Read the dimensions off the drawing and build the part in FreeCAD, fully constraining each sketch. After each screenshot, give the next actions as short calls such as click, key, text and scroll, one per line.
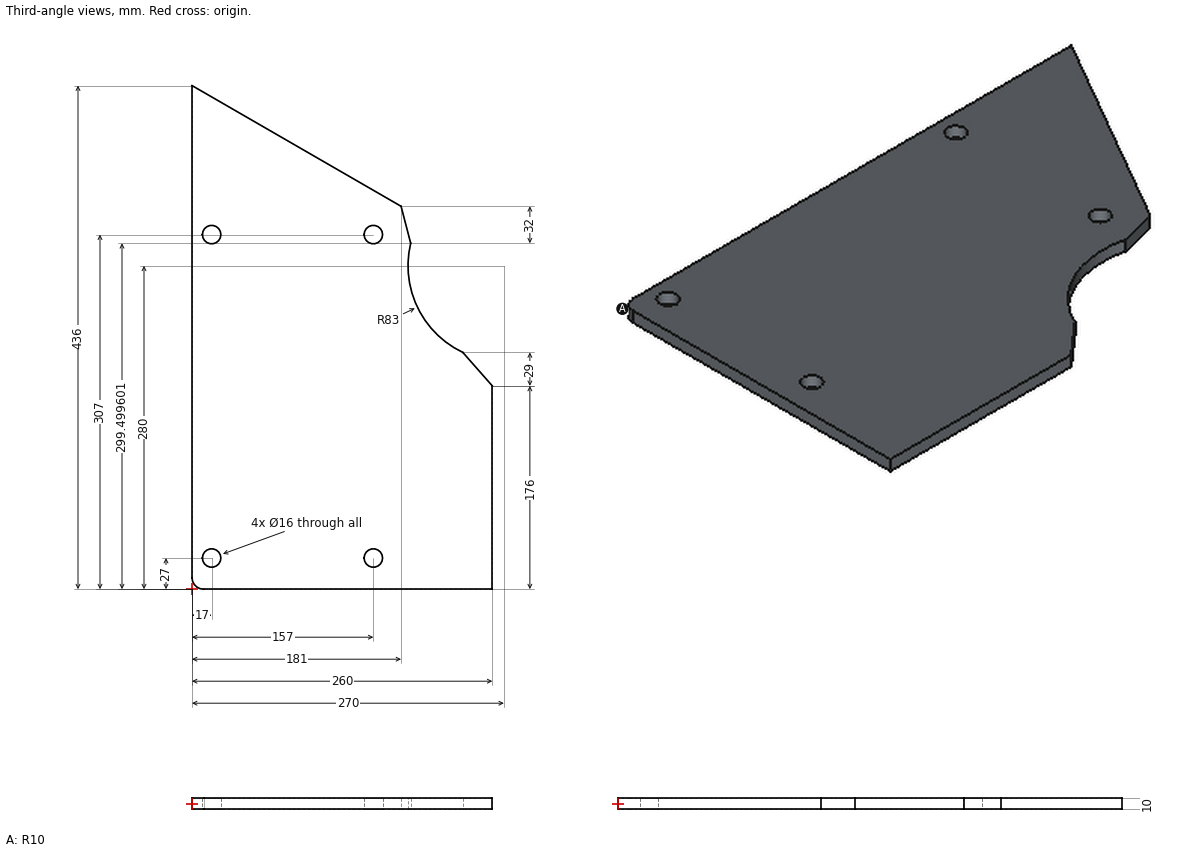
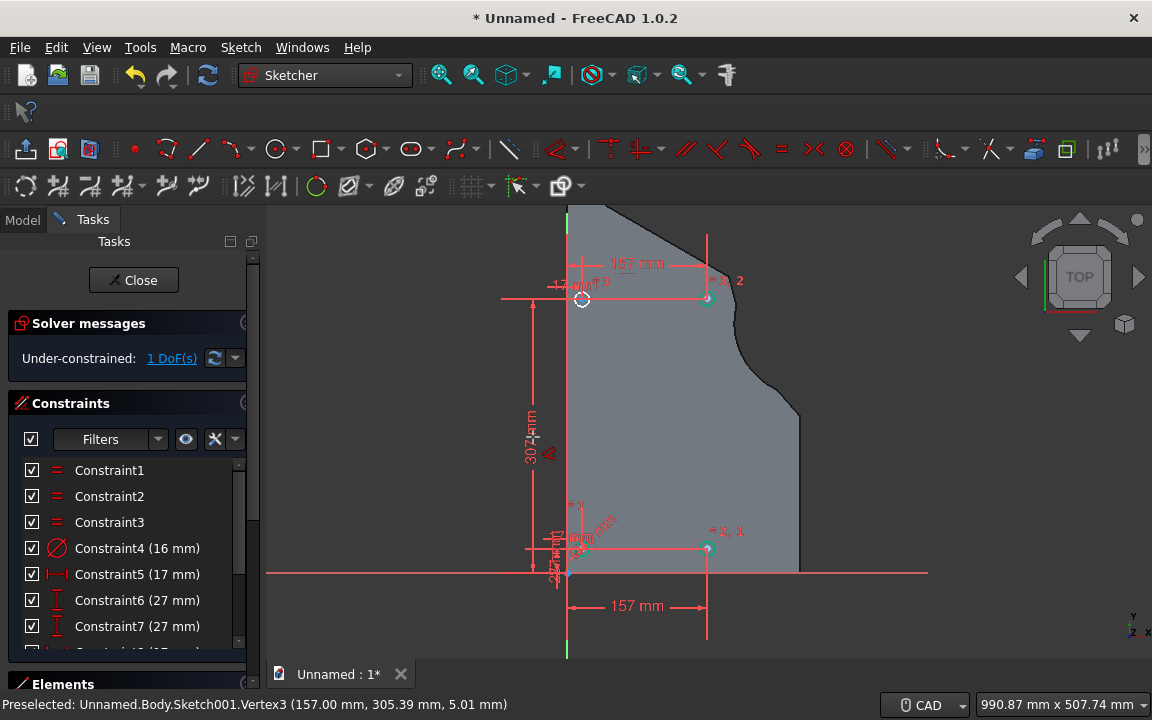
click(582, 299)
click(533, 373)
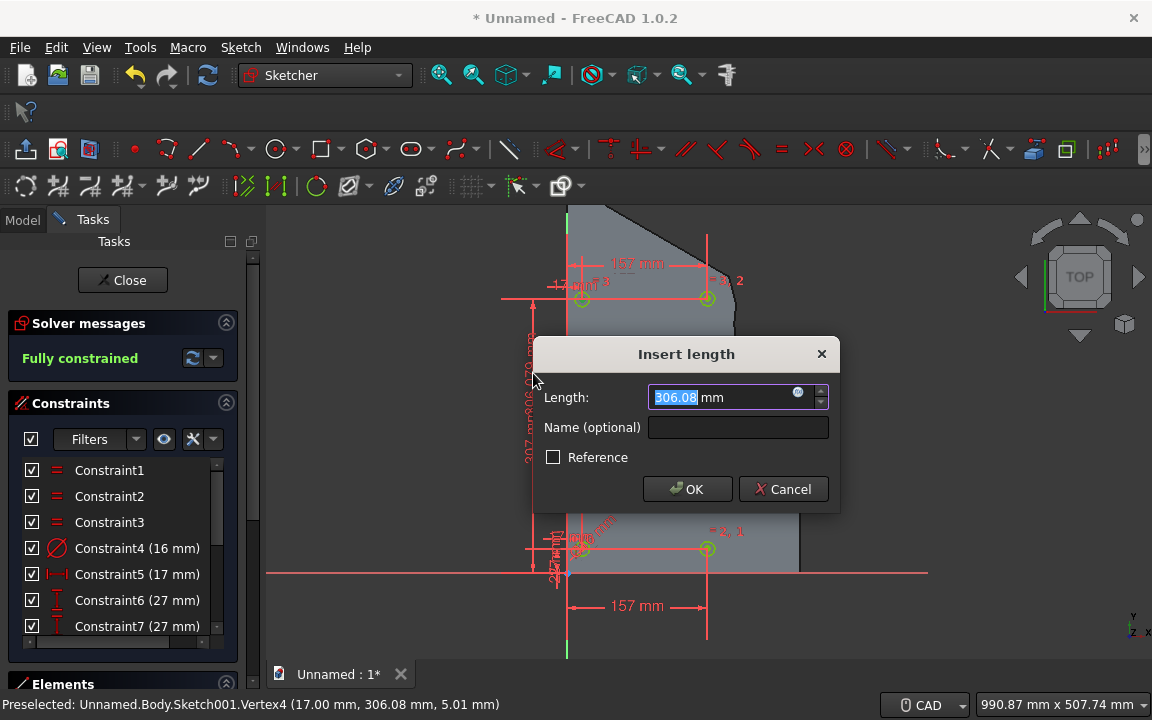
text(307)
key(Return)
key(Escape)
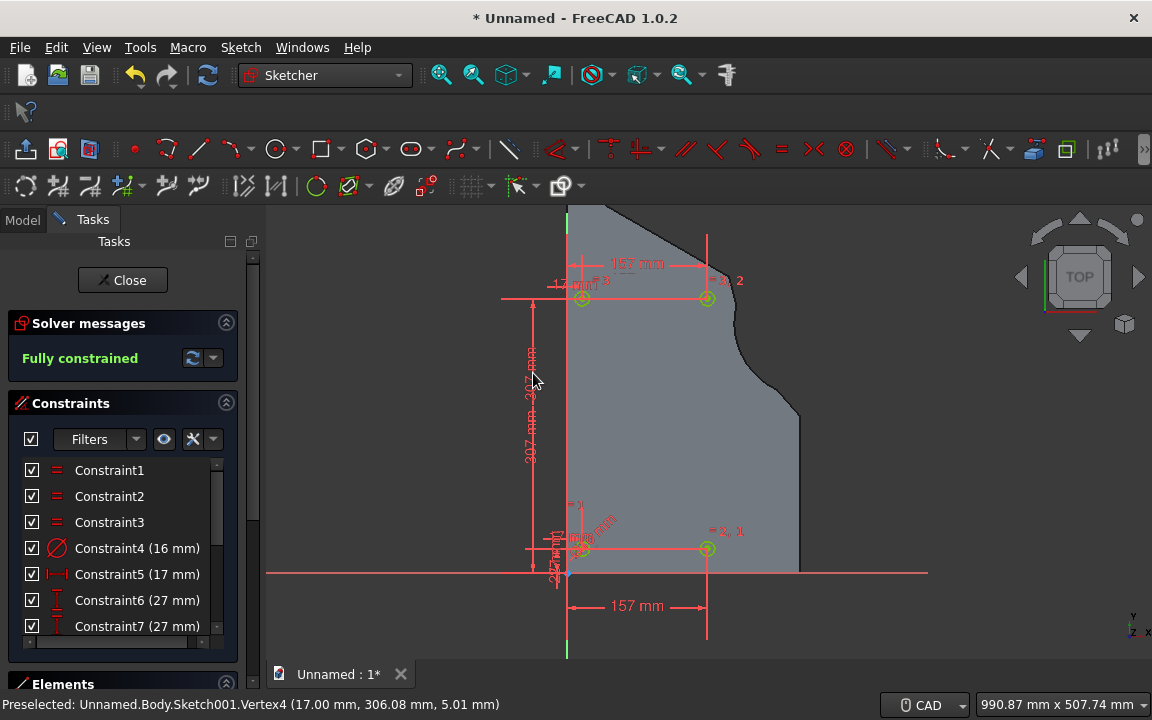
click(123, 280)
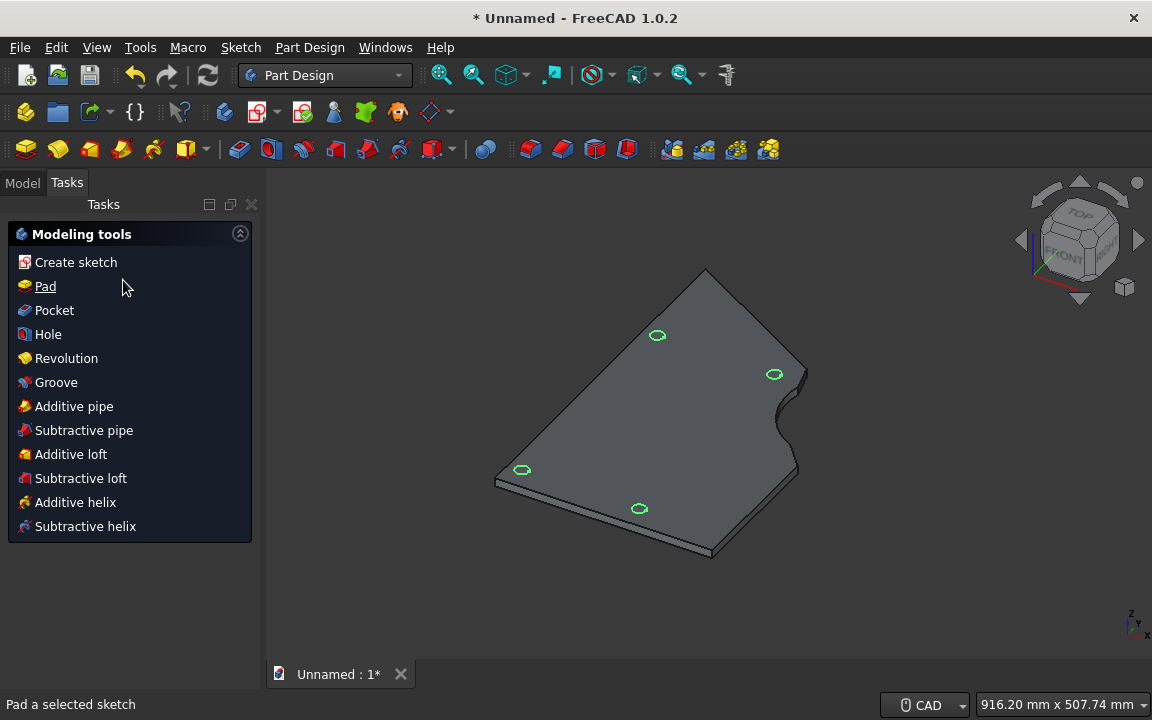
click(272, 150)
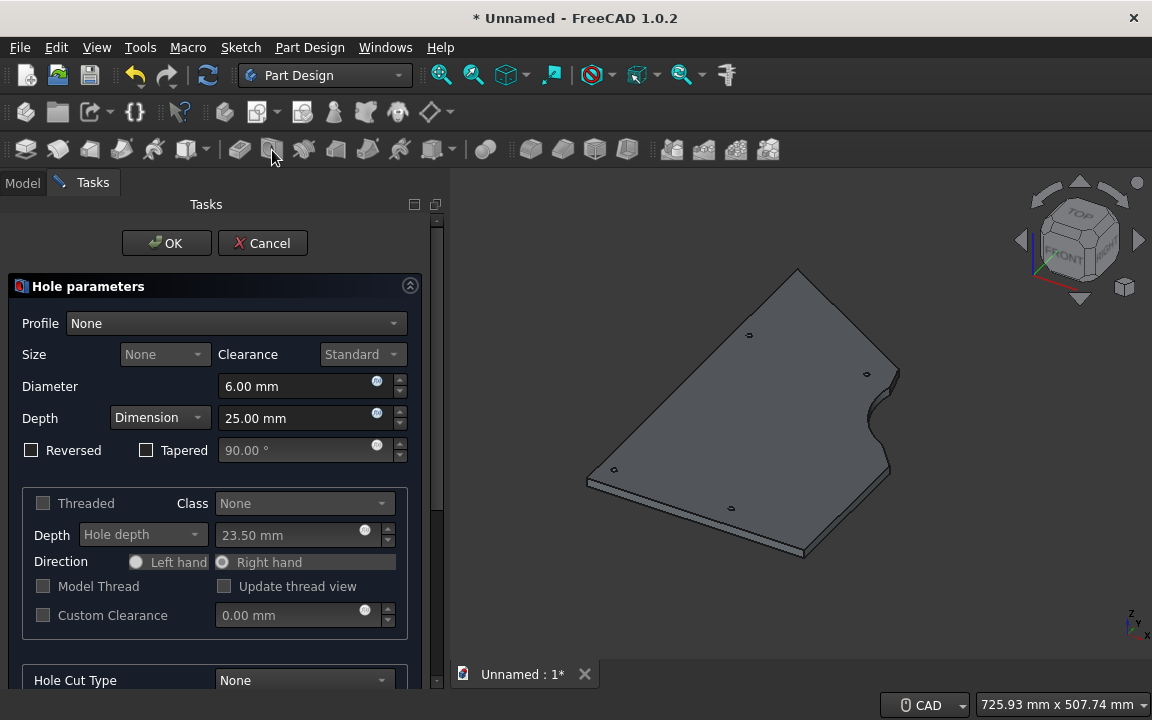
triple_click(305, 386)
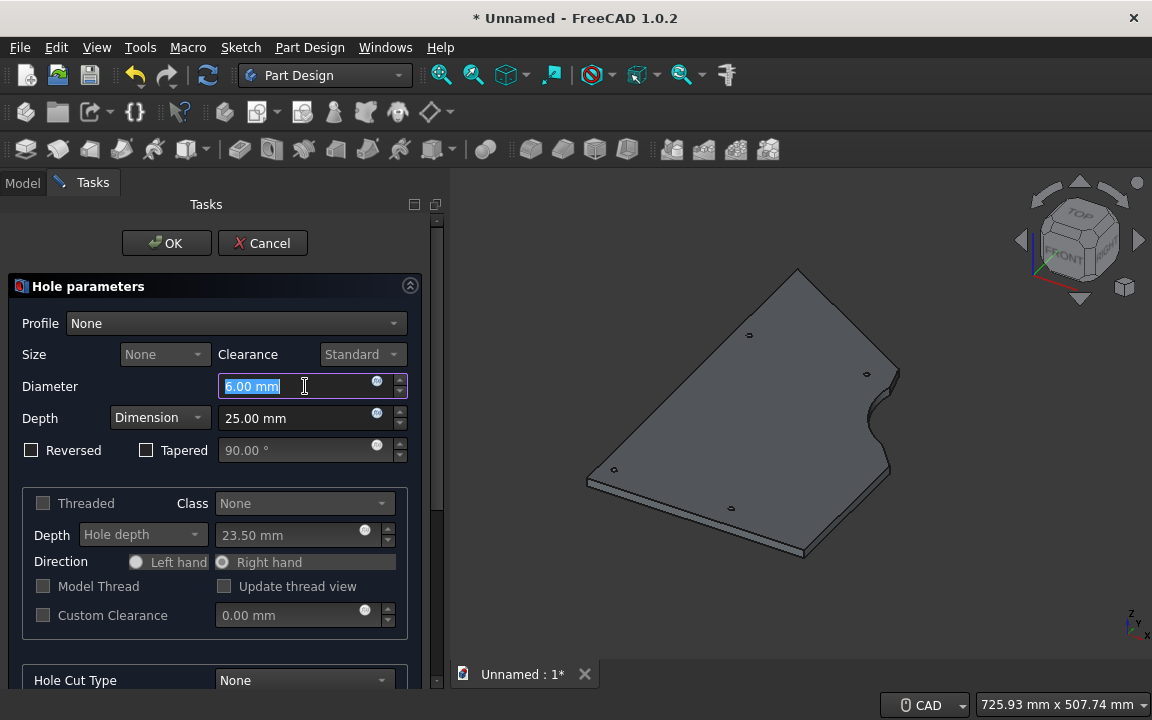
text(16)
key(Tab)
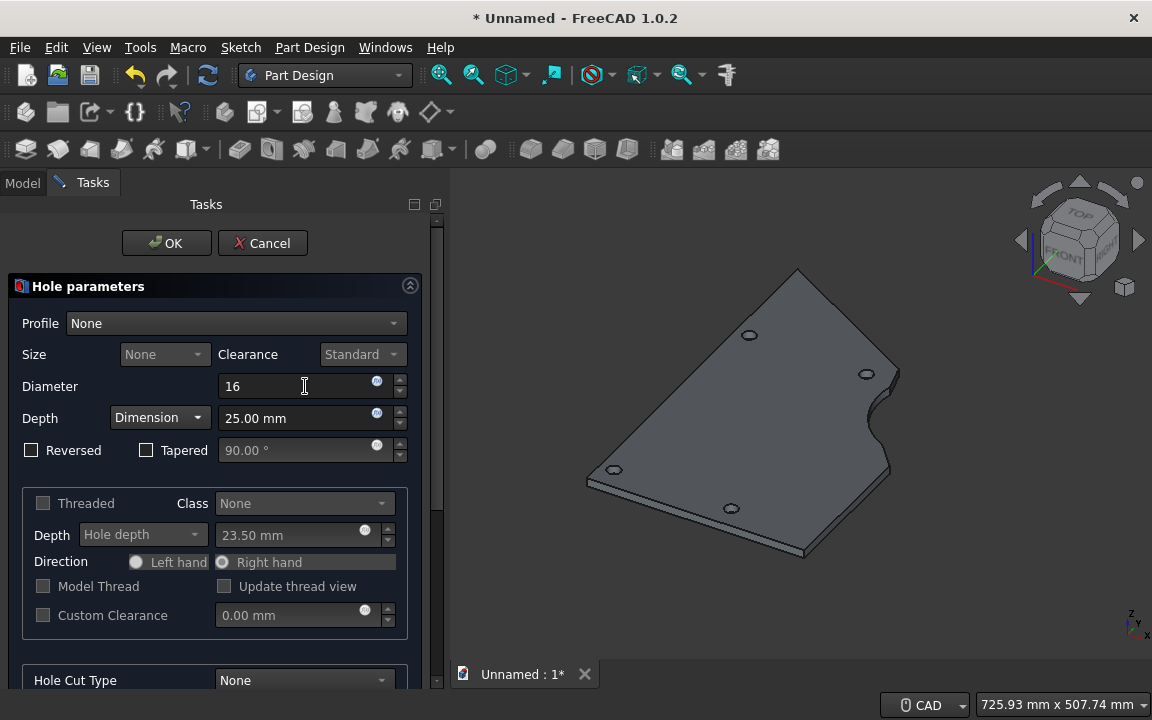
click(161, 418)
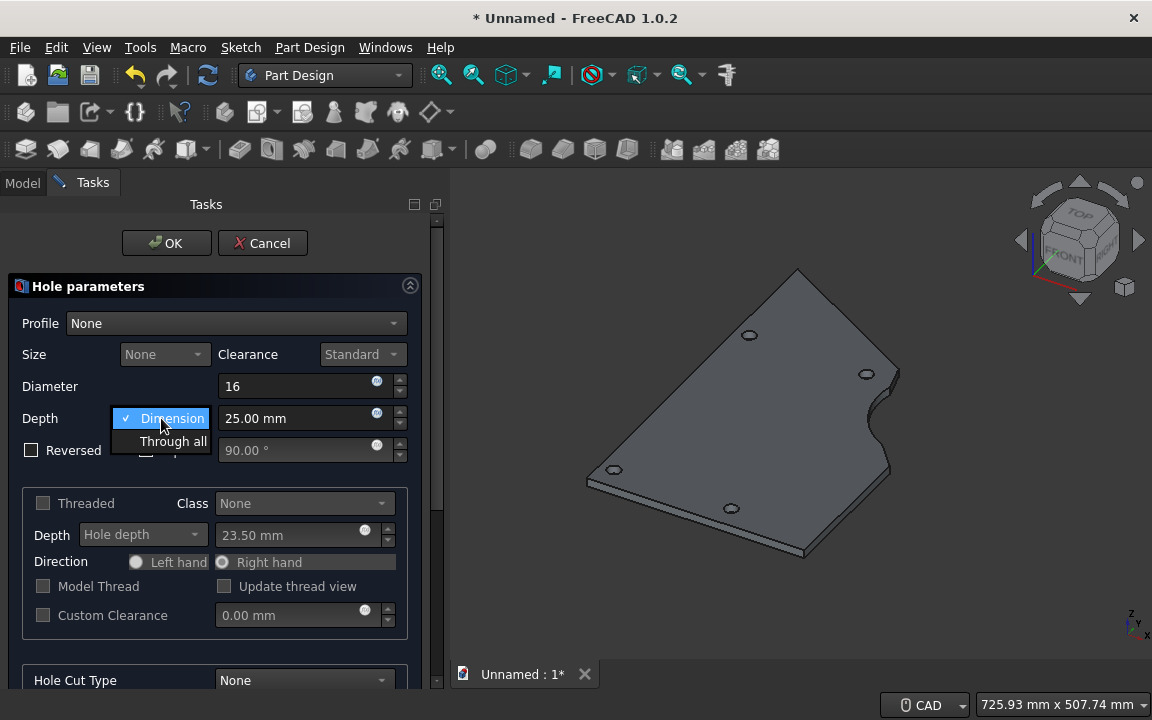
click(160, 442)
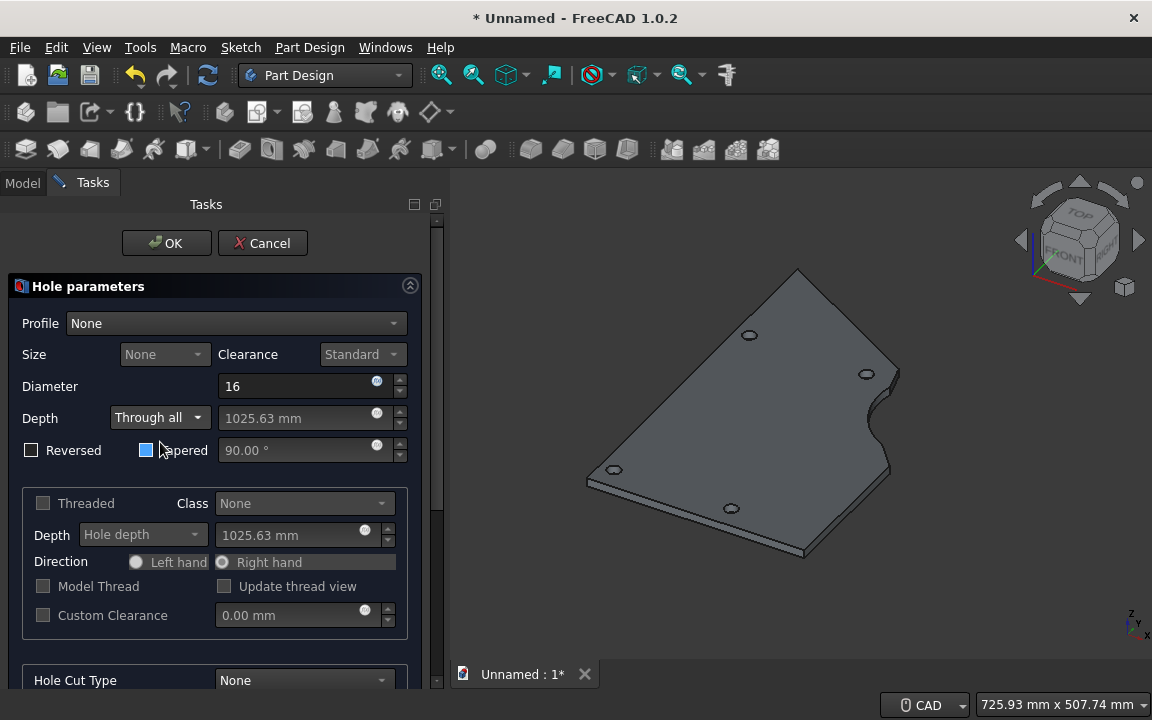
click(167, 243)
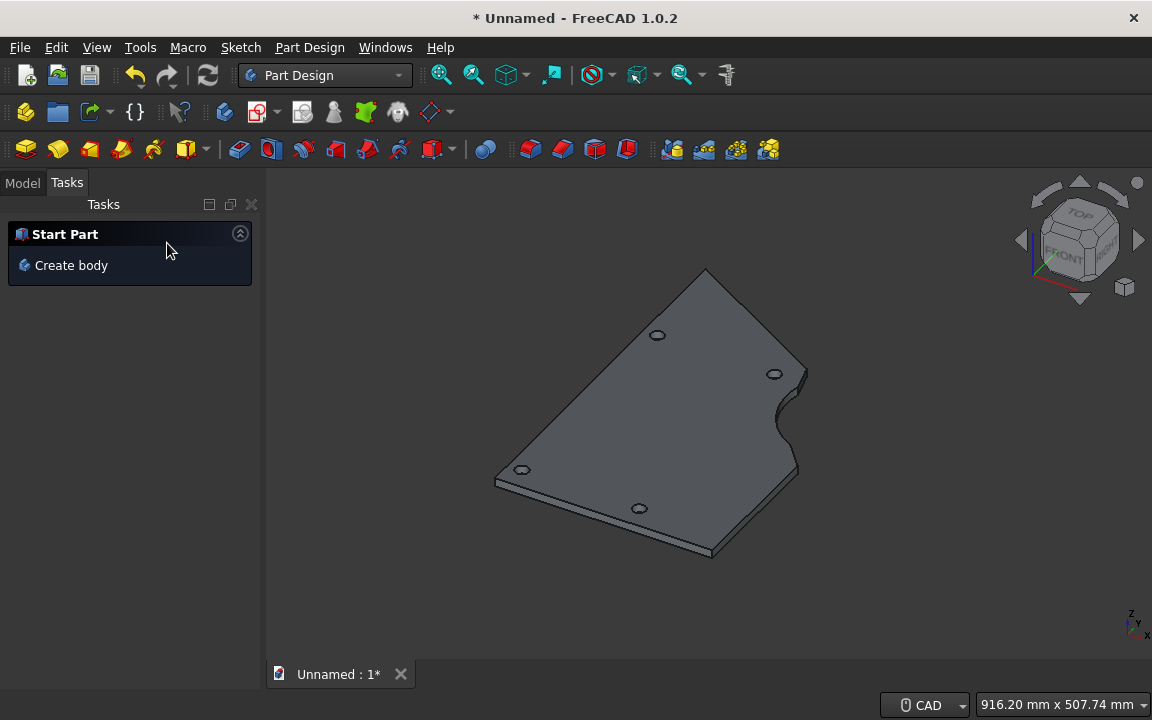
scroll(495, 481, up, 8)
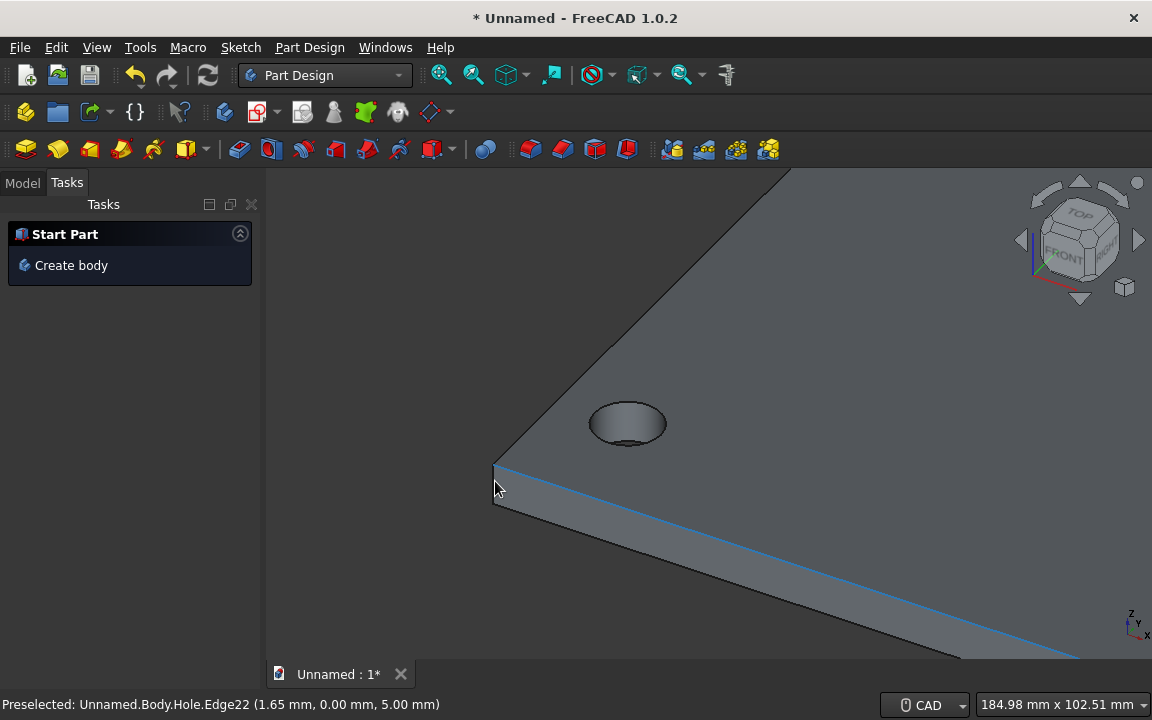
key(v)
key(f)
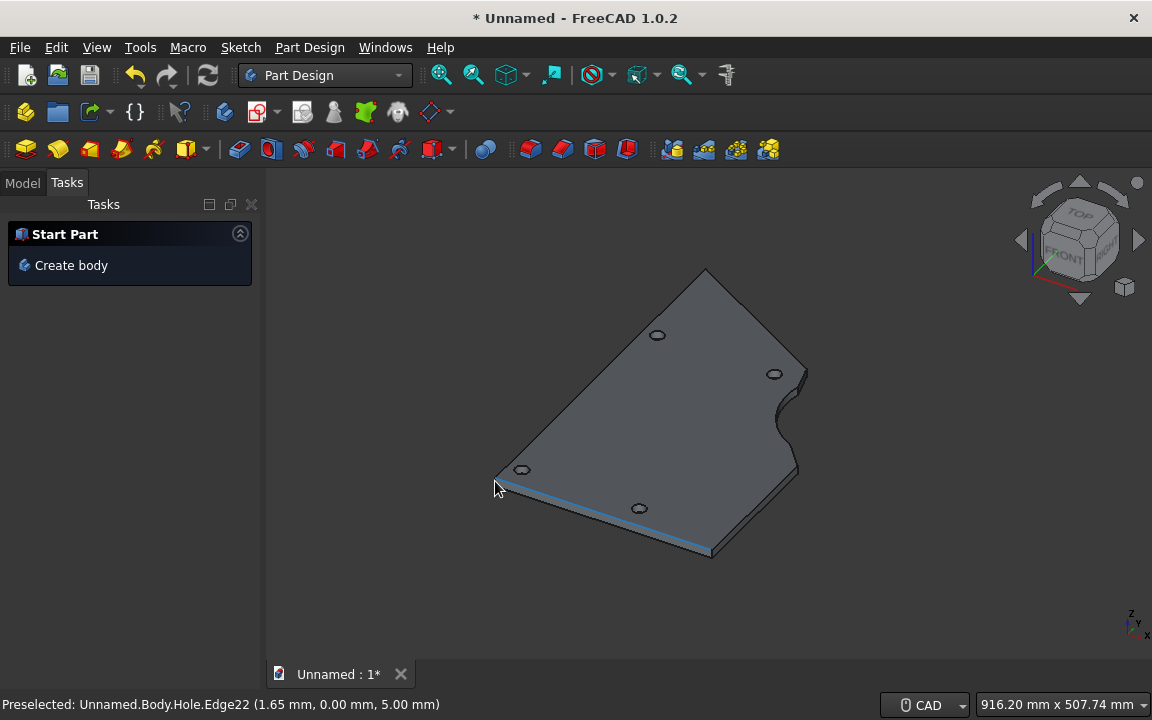
key(0)